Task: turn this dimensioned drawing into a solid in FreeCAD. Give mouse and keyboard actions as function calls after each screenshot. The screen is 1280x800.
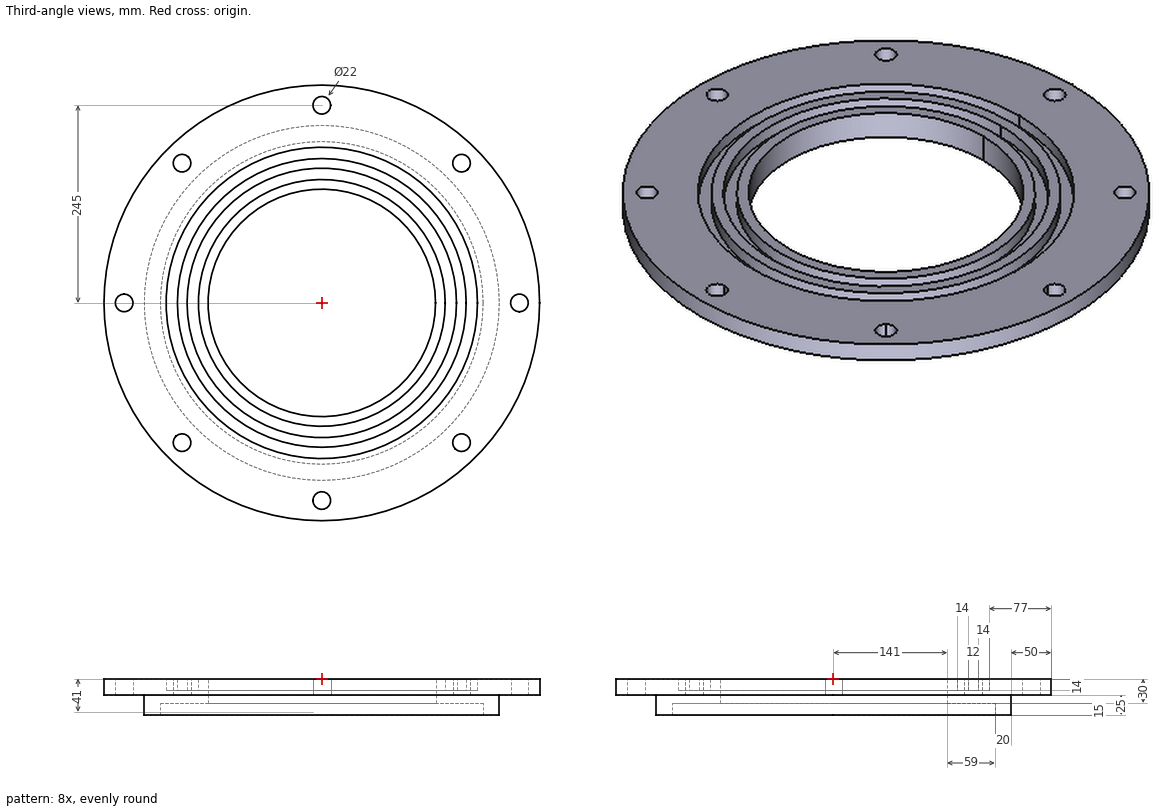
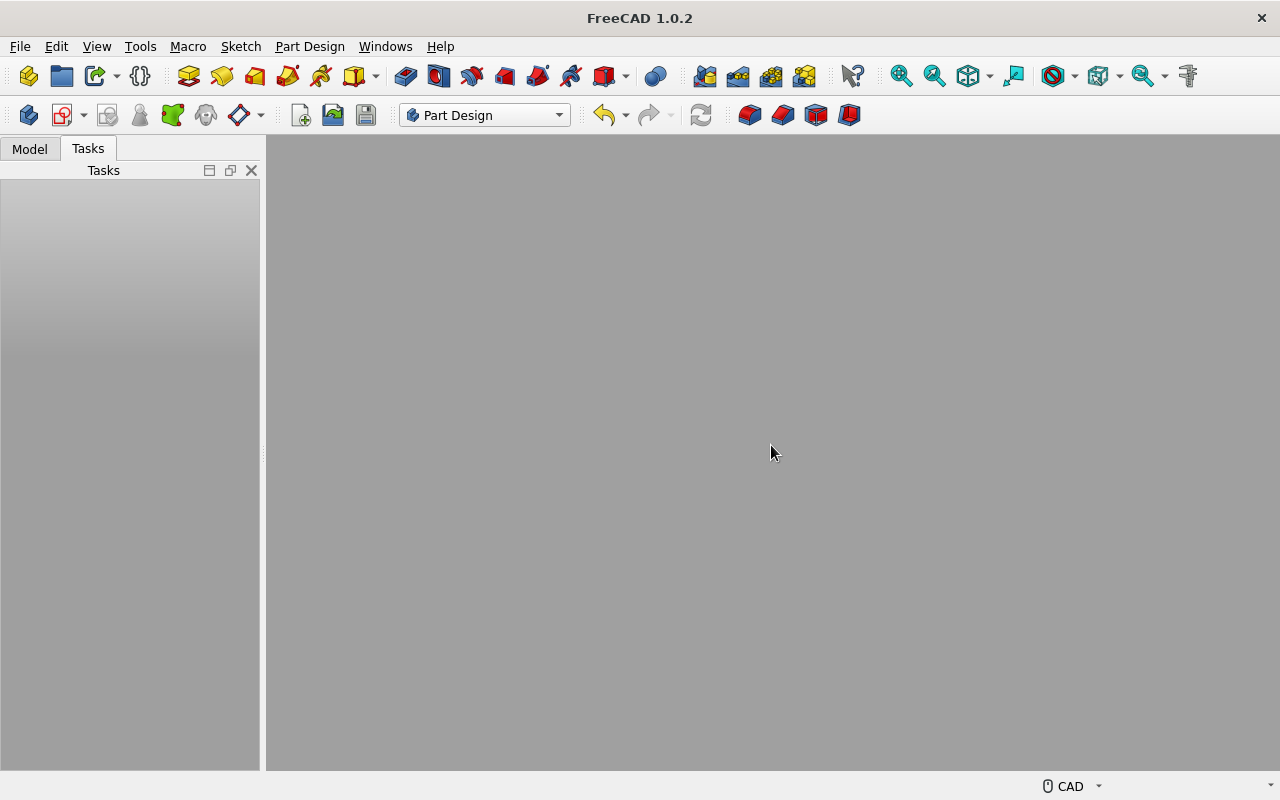
click(300, 116)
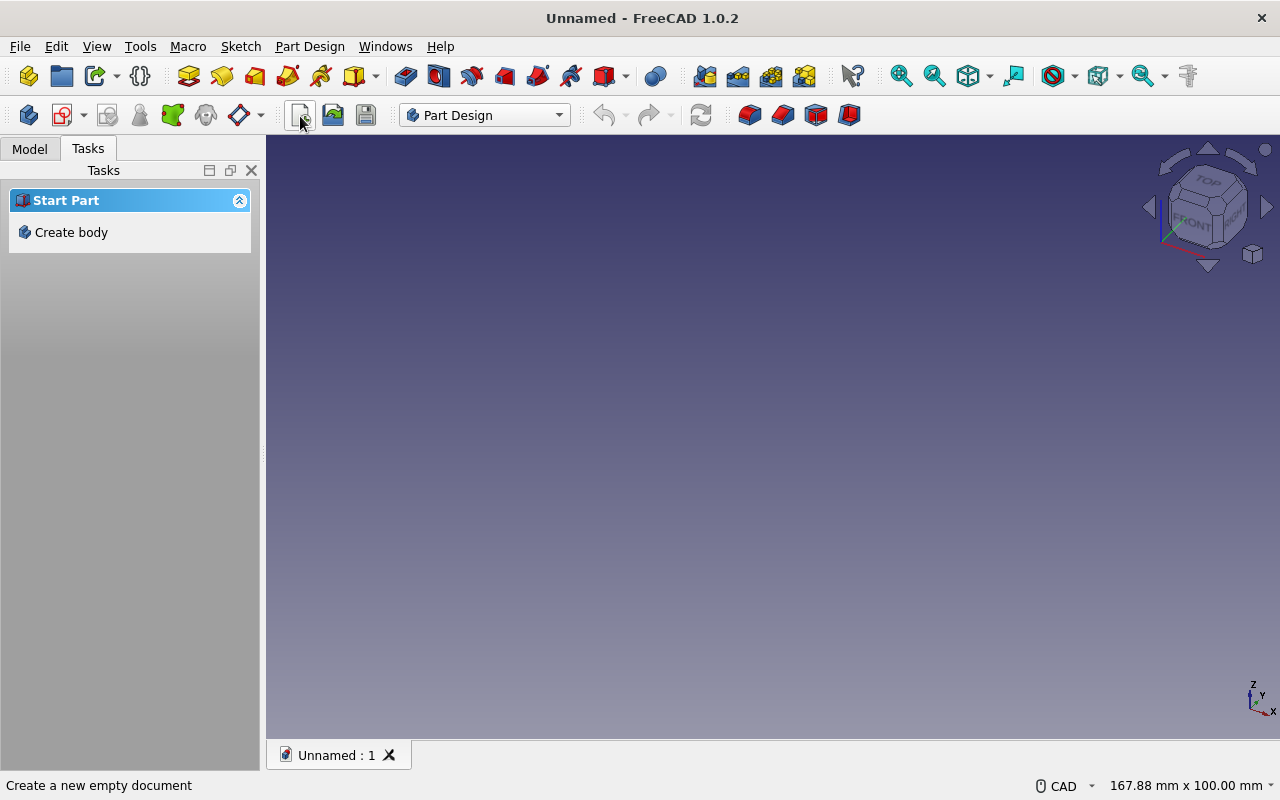
click(62, 116)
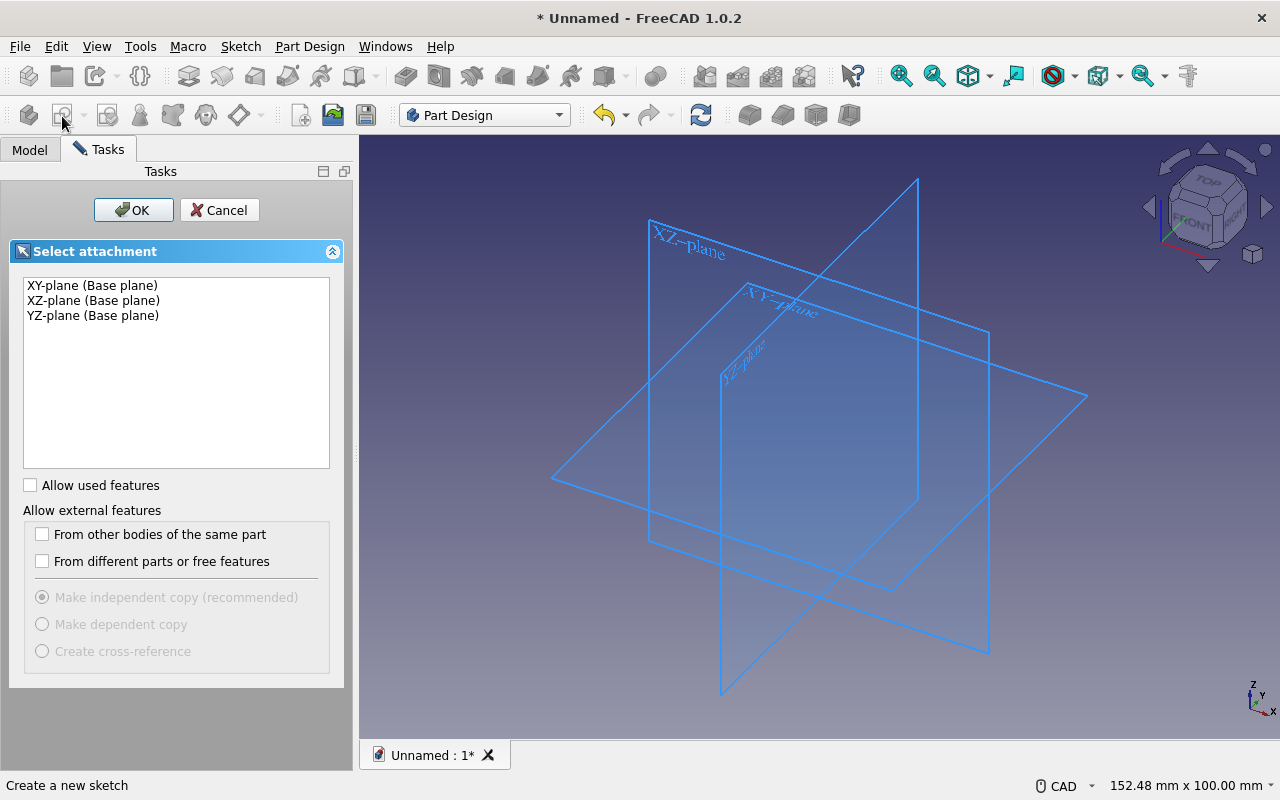
click(84, 316)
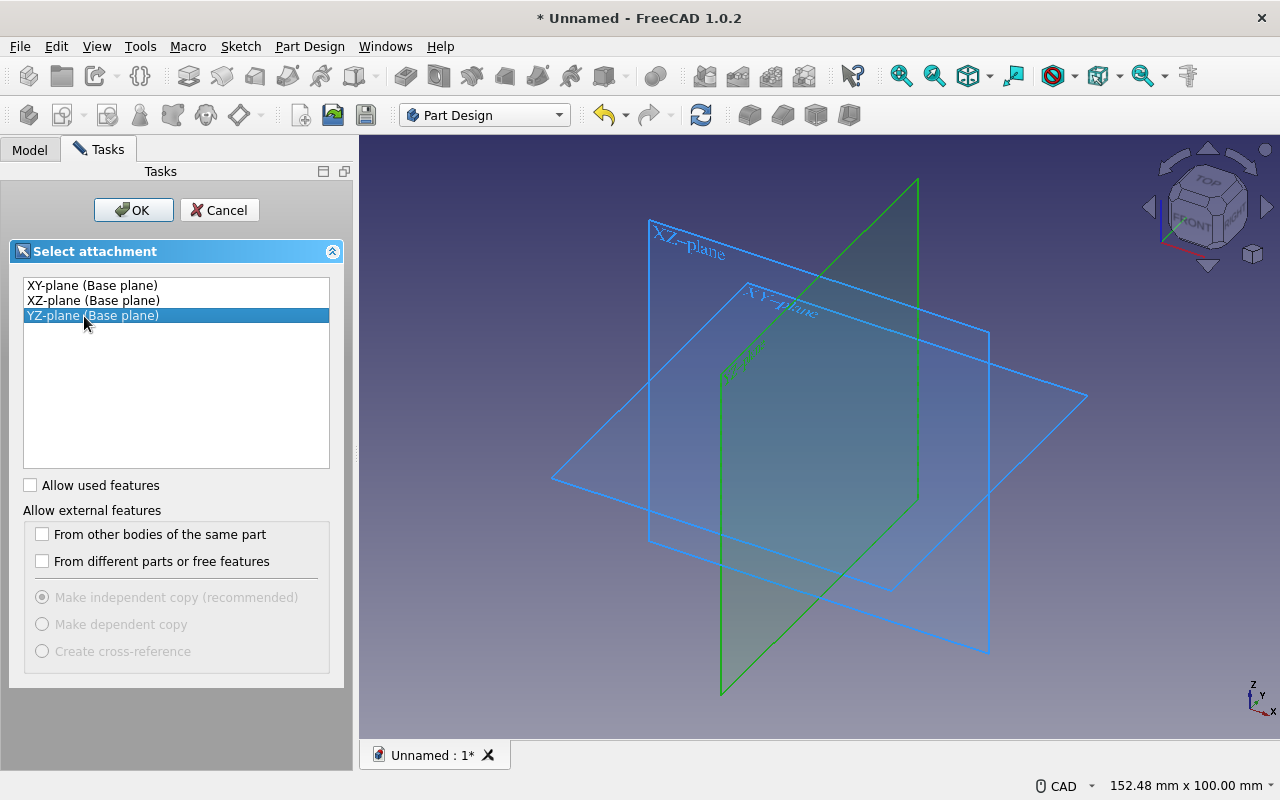
click(134, 210)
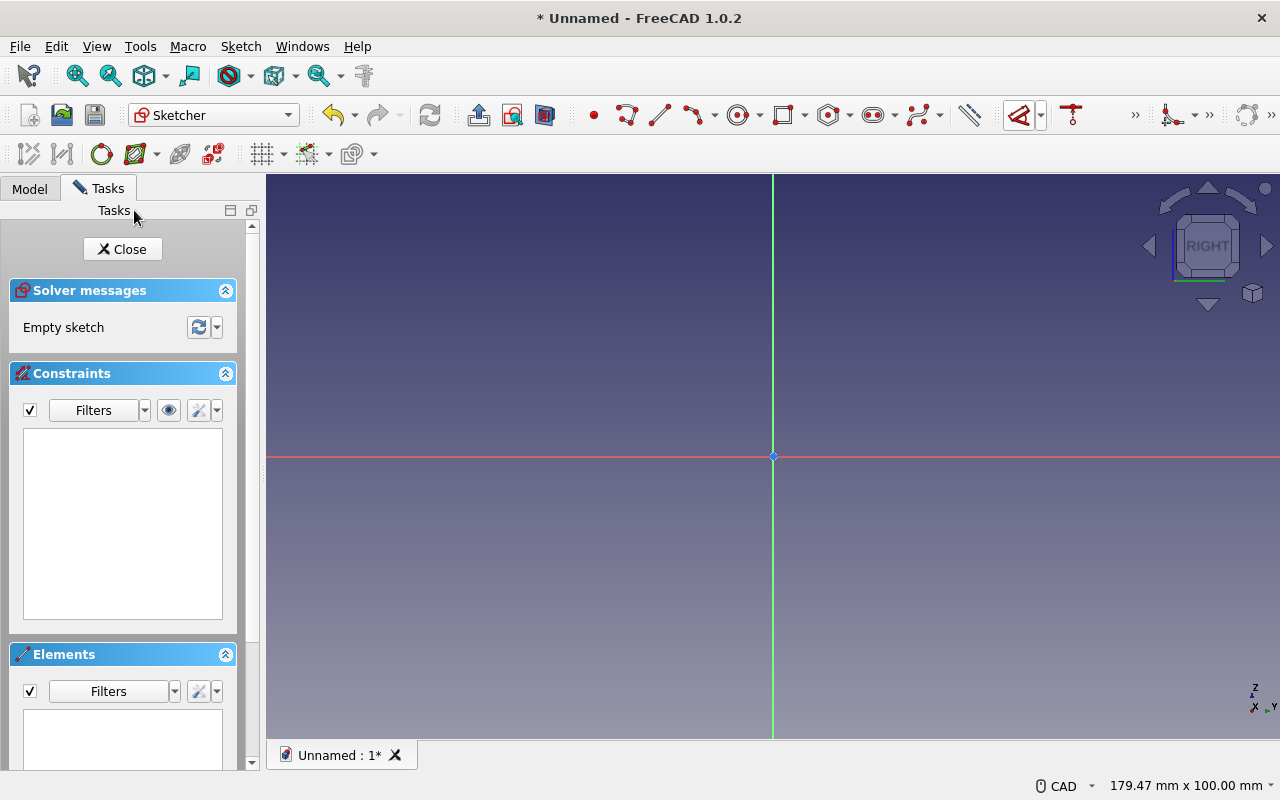
scroll(294, 383, down, 5)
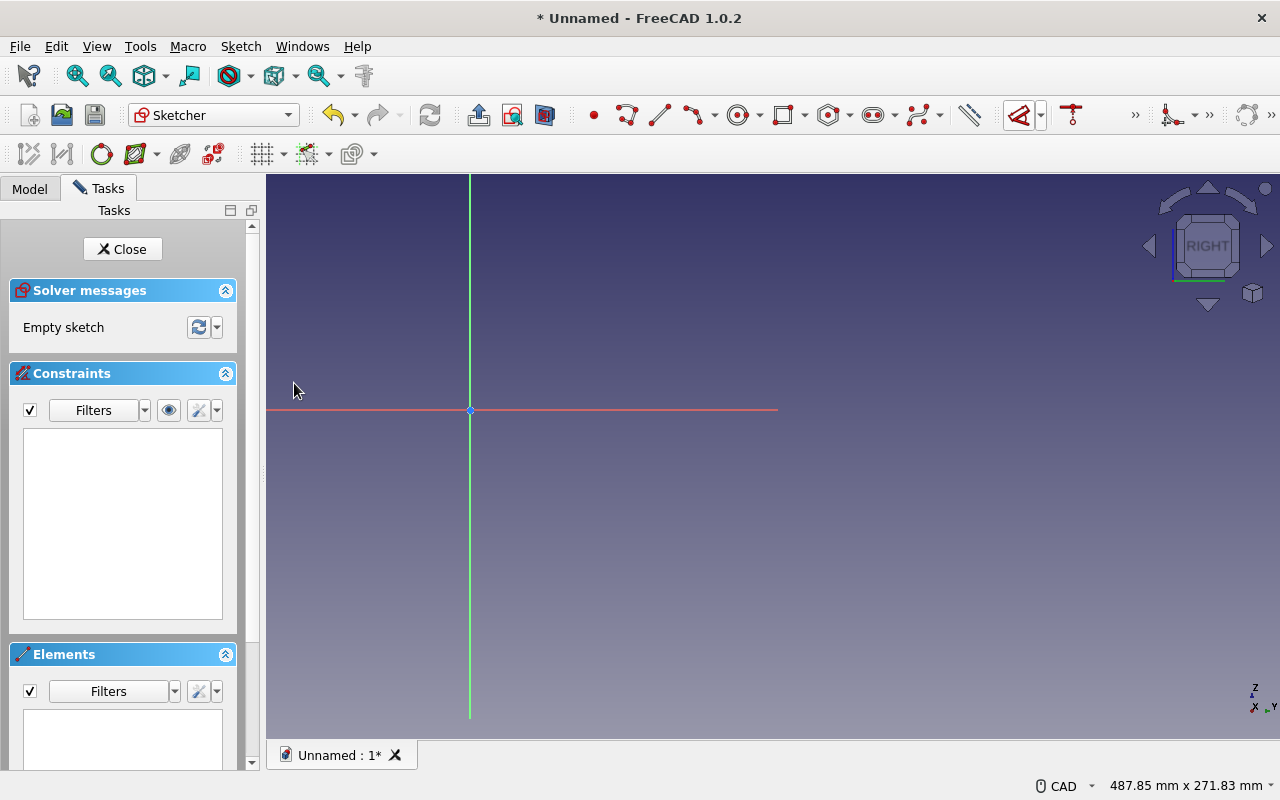
click(627, 116)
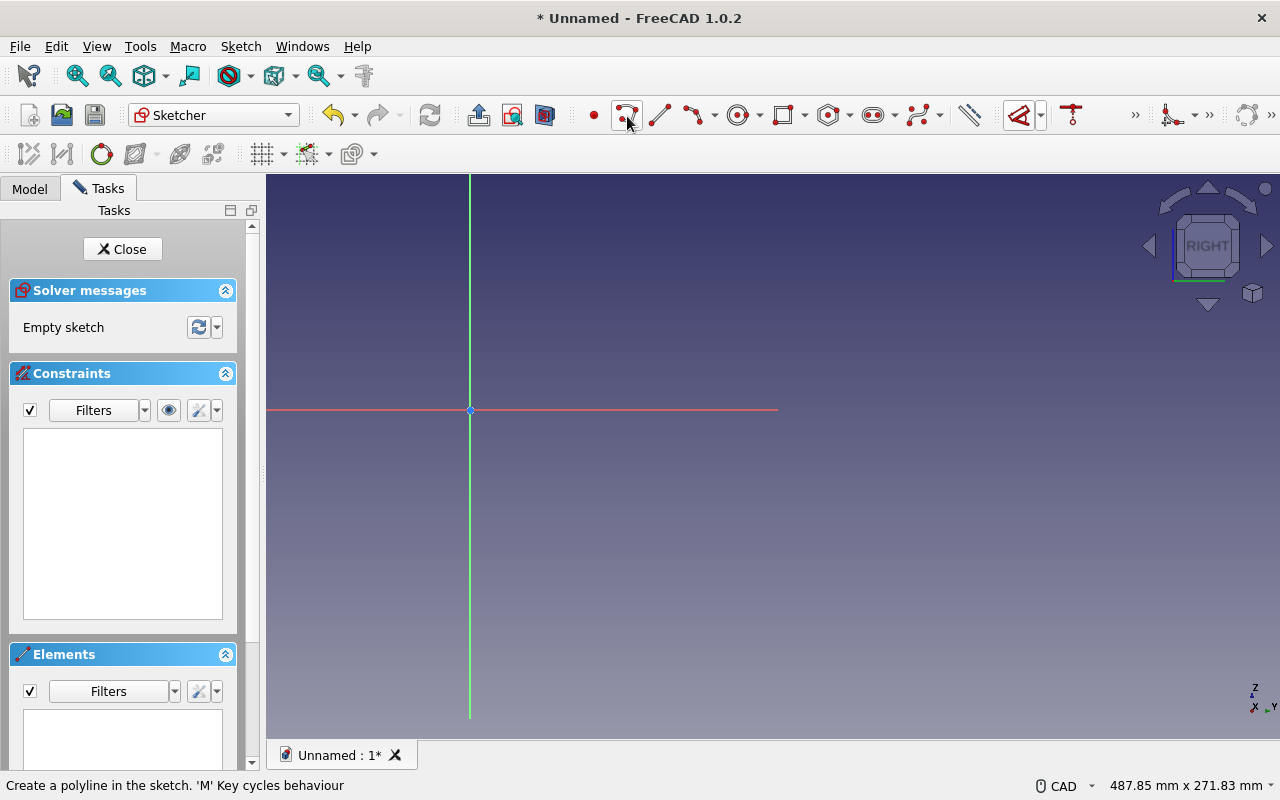
click(763, 410)
click(763, 473)
click(886, 473)
click(886, 504)
click(928, 504)
click(928, 452)
click(1031, 452)
click(1031, 410)
click(871, 419)
click(871, 439)
click(842, 439)
click(842, 410)
click(817, 419)
click(817, 439)
click(788, 439)
click(788, 419)
click(763, 410)
key(Escape)
key(Escape)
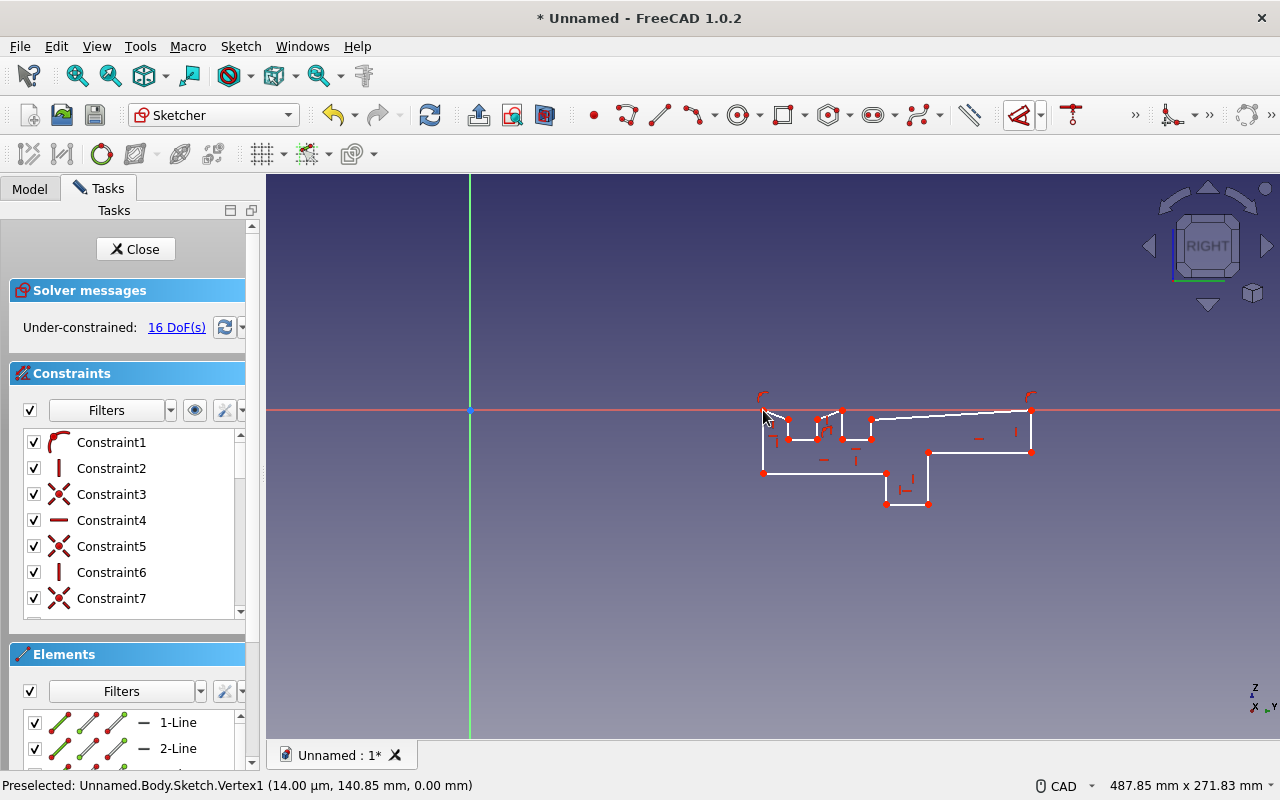
click(983, 413)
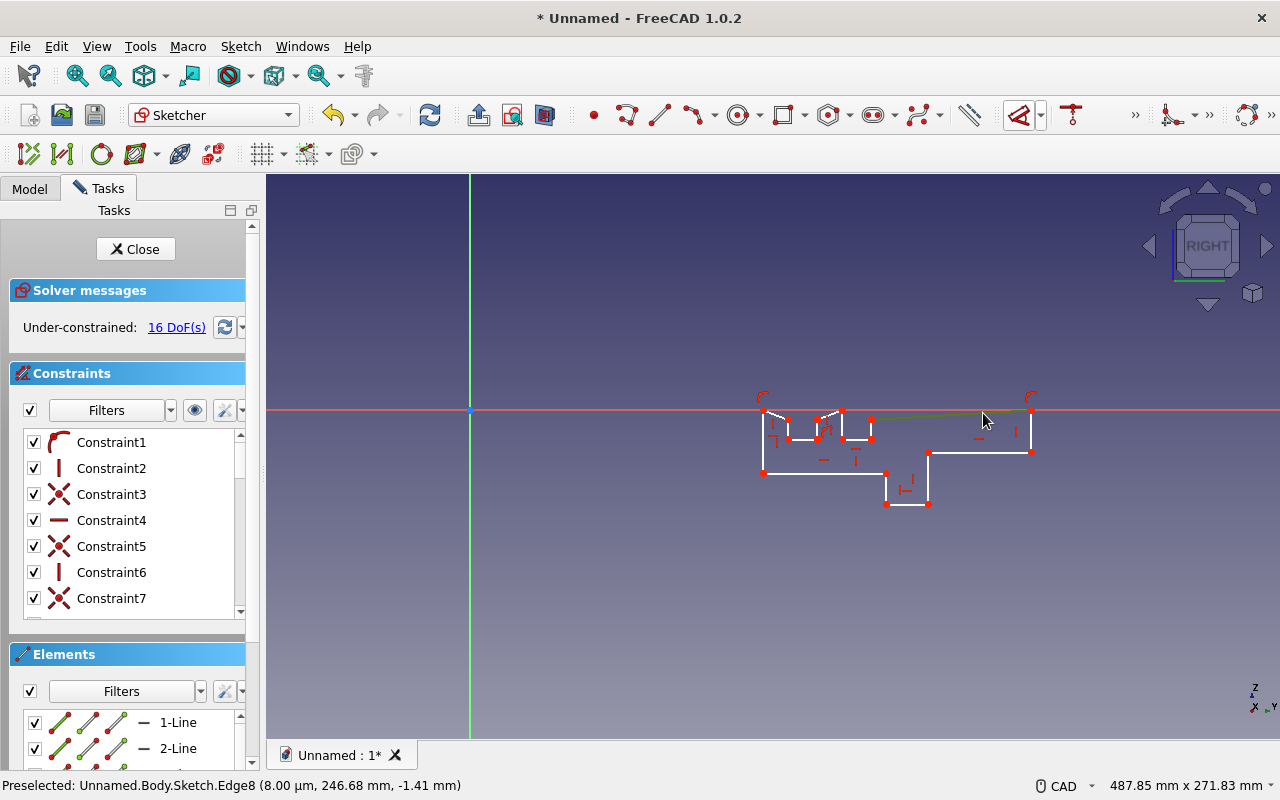
key(h)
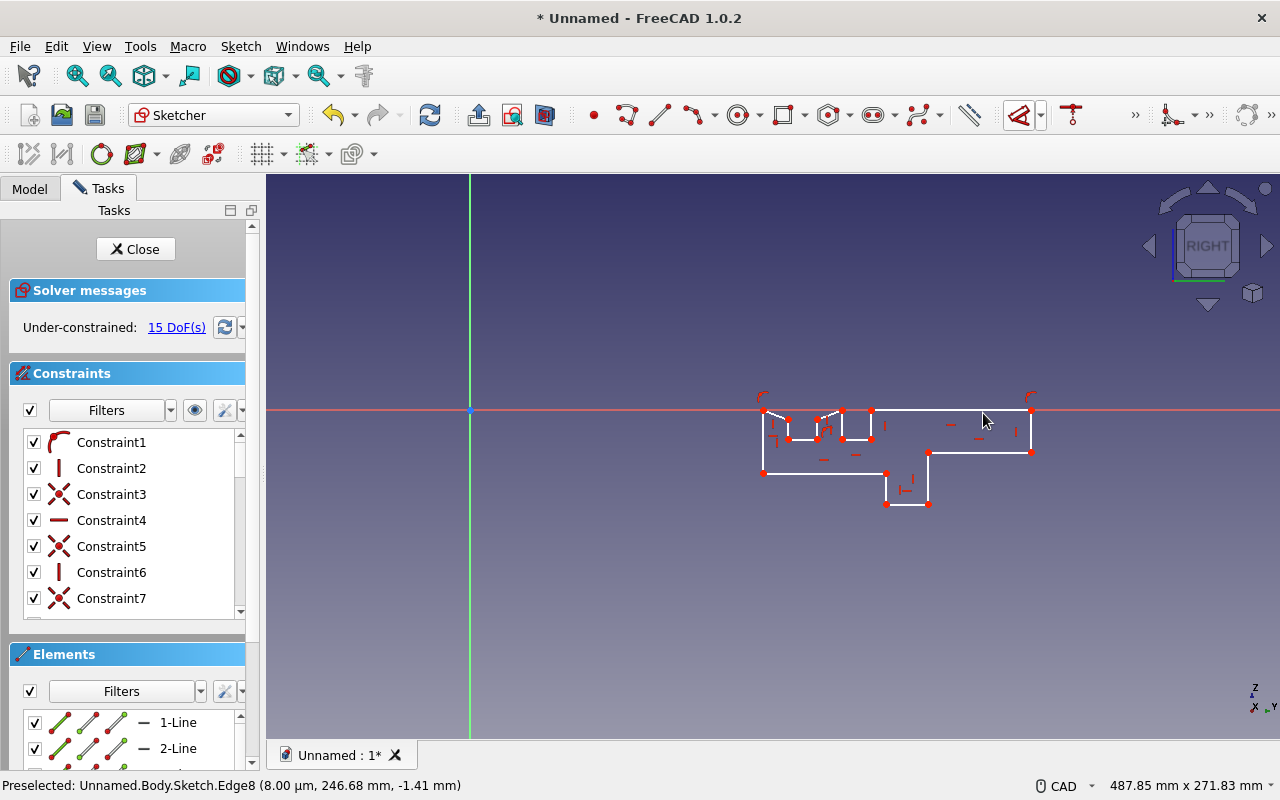
scroll(832, 414, up, 2)